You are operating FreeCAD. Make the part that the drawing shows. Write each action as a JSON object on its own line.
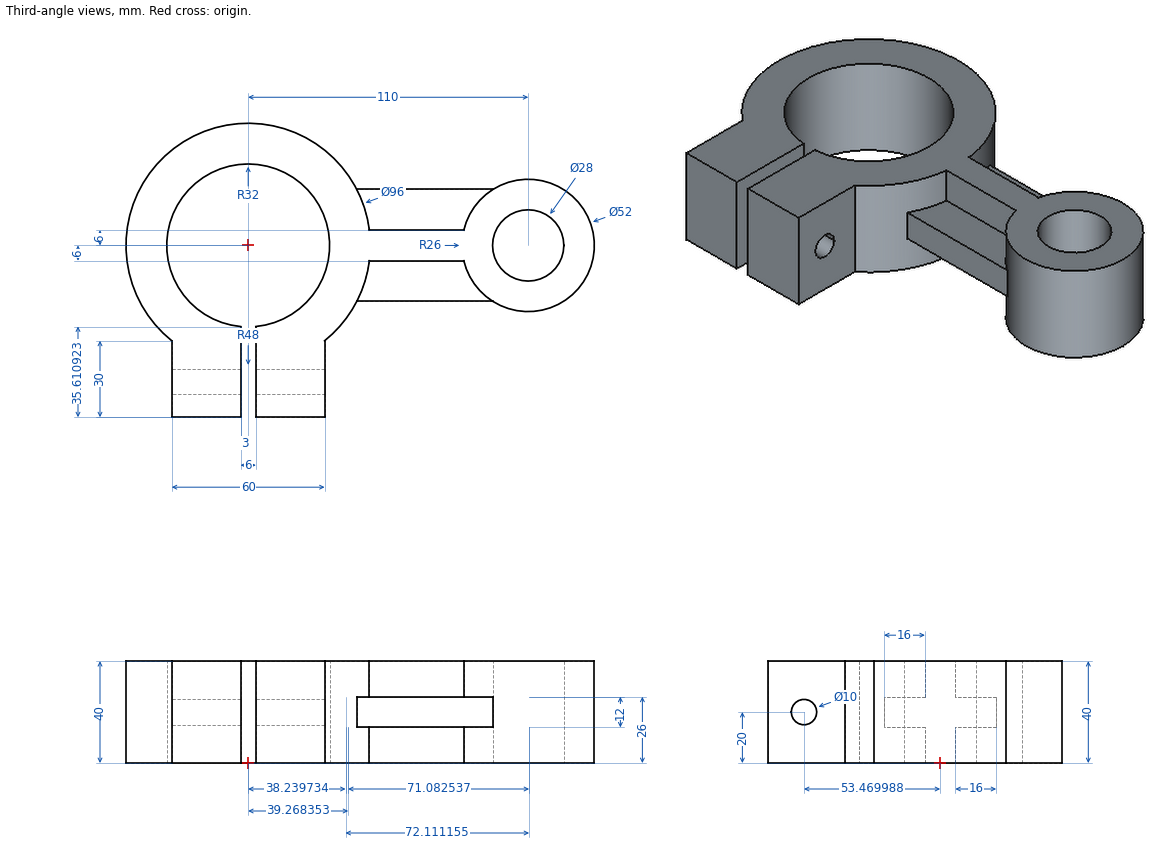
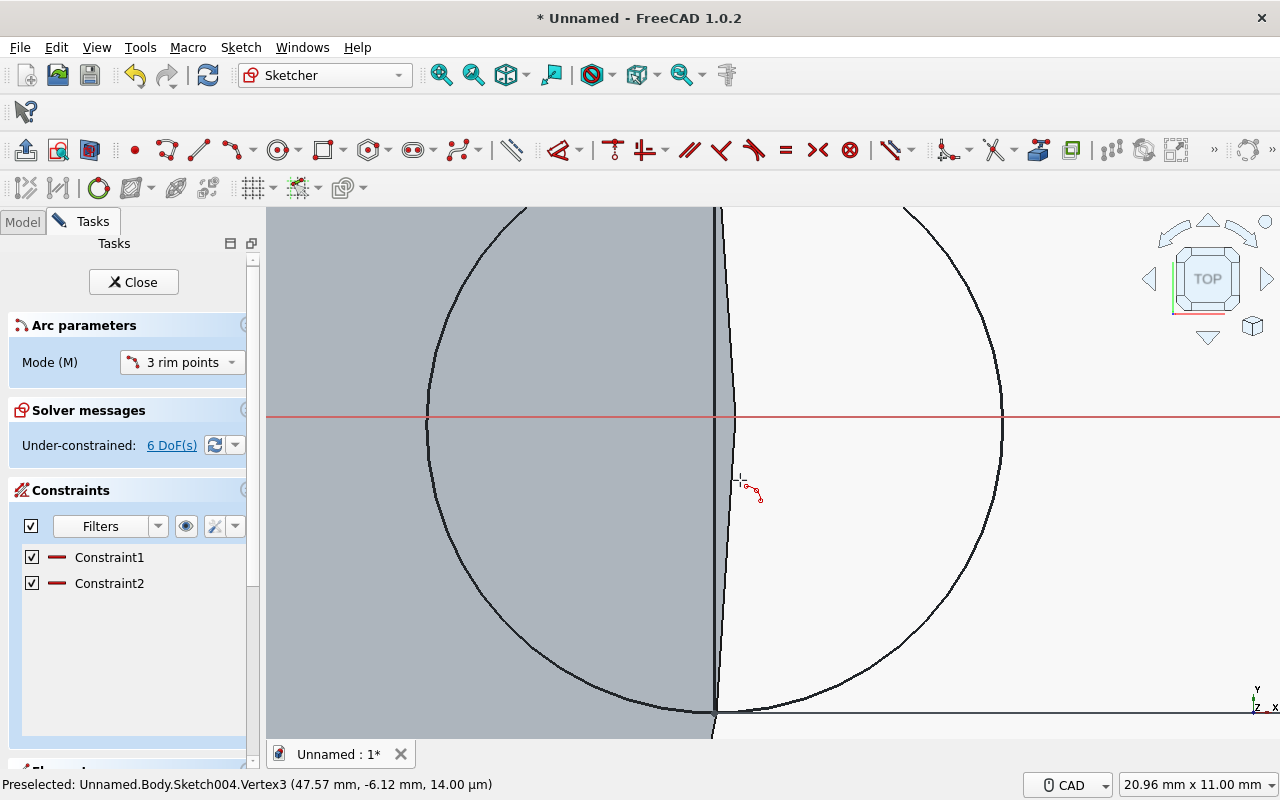
{"action": "left_click", "coordinate": [735, 475]}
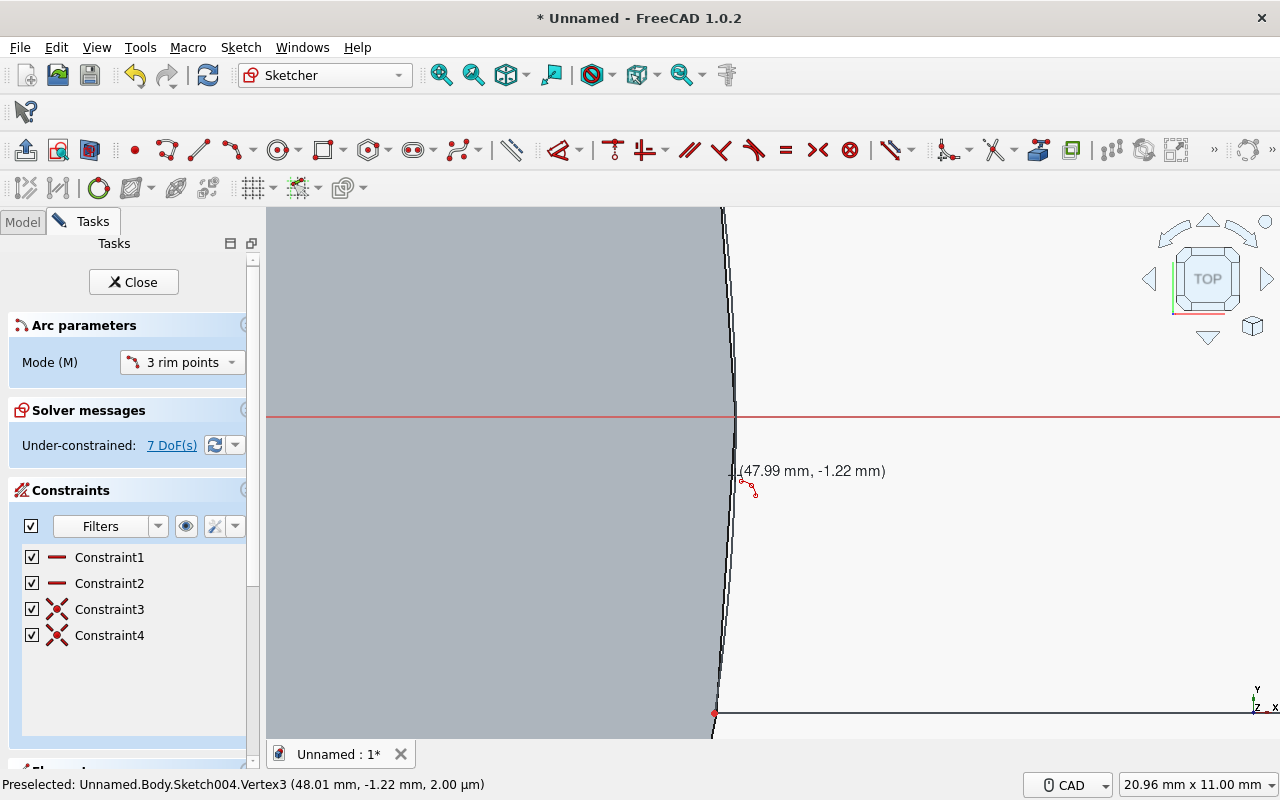
{"action": "scroll", "coordinate": [742, 482], "scroll_direction": "down", "scroll_amount": 10}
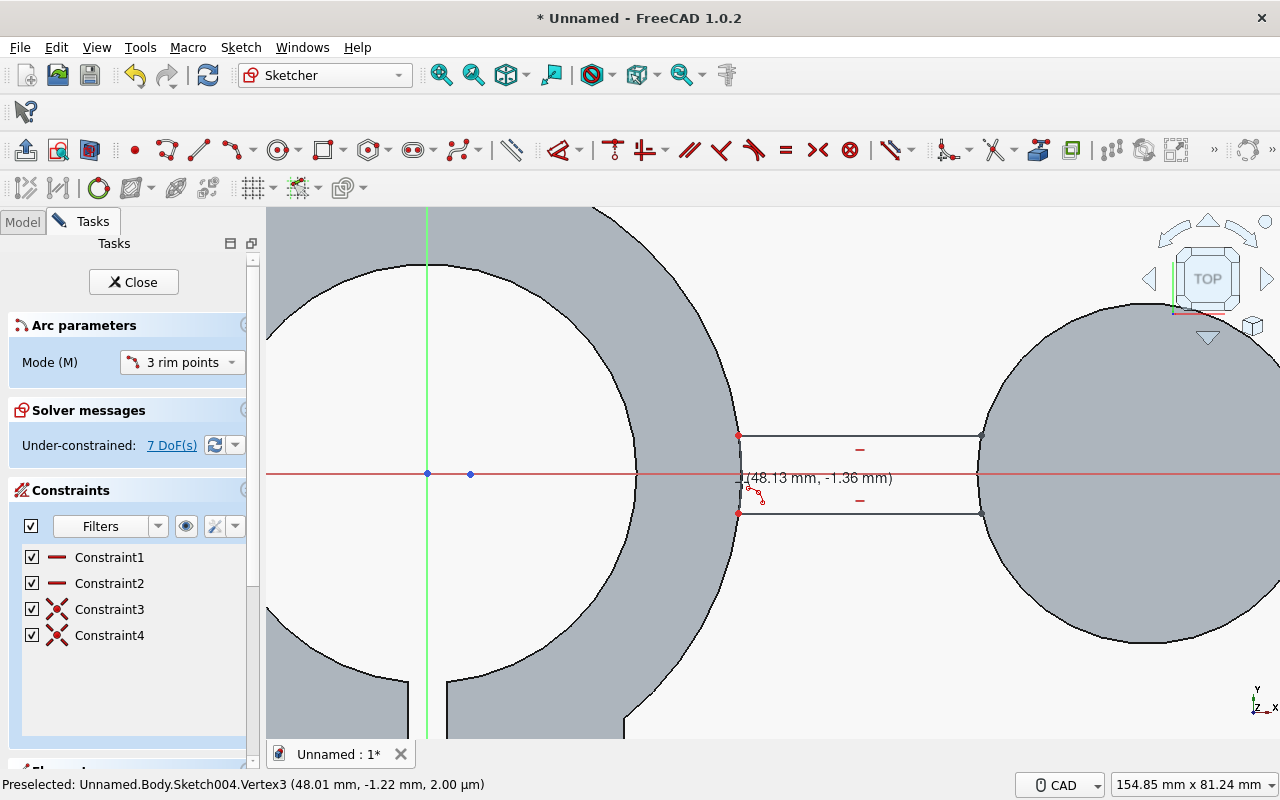
{"action": "left_click", "coordinate": [982, 514]}
{"action": "left_click", "coordinate": [982, 436]}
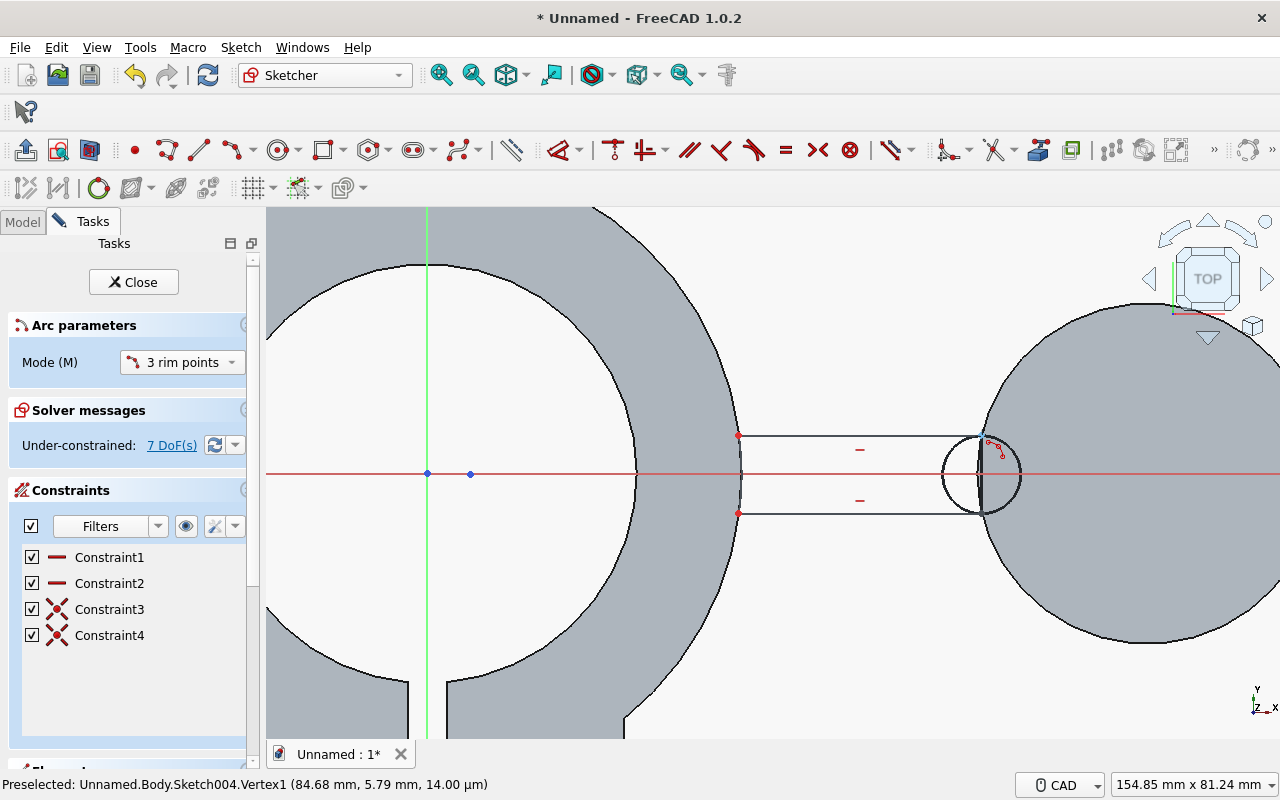
{"action": "scroll", "coordinate": [977, 466], "scroll_direction": "up", "scroll_amount": 7}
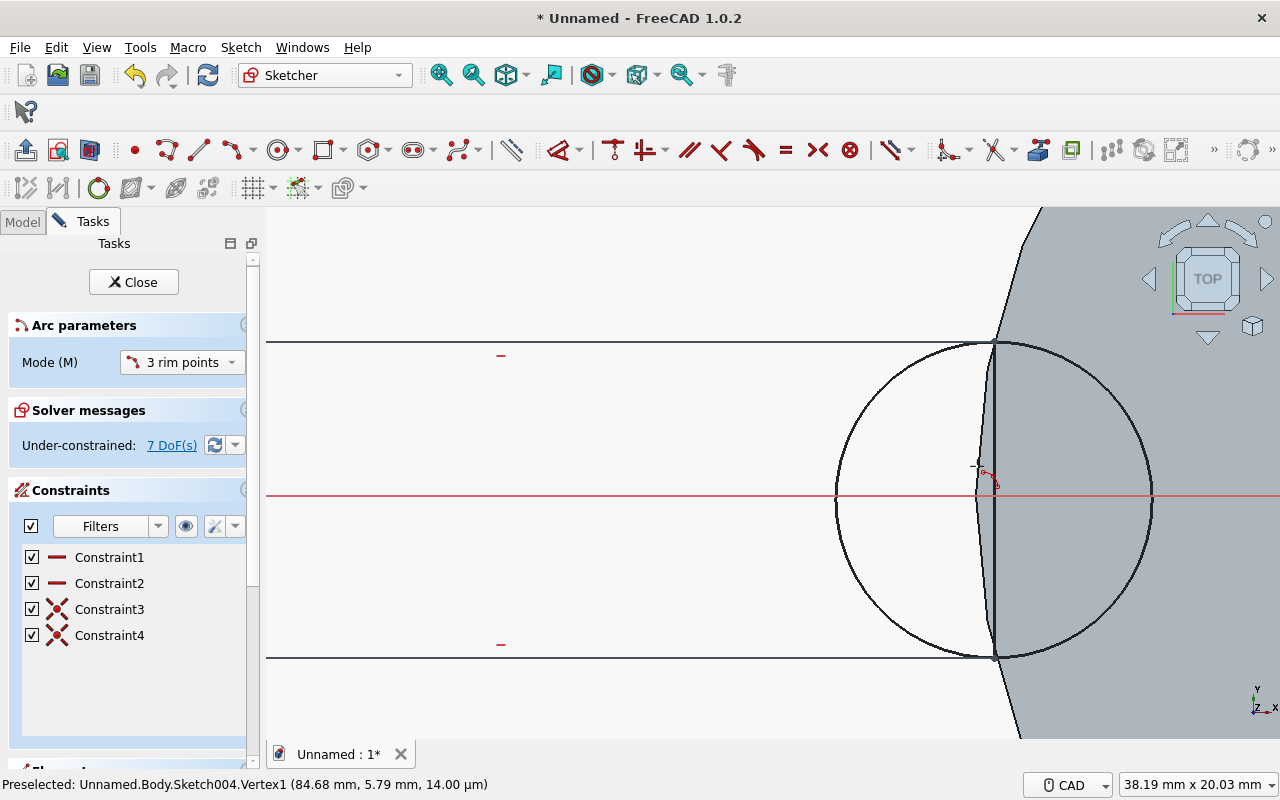
{"action": "left_click", "coordinate": [977, 463]}
{"action": "key", "text": "Escape"}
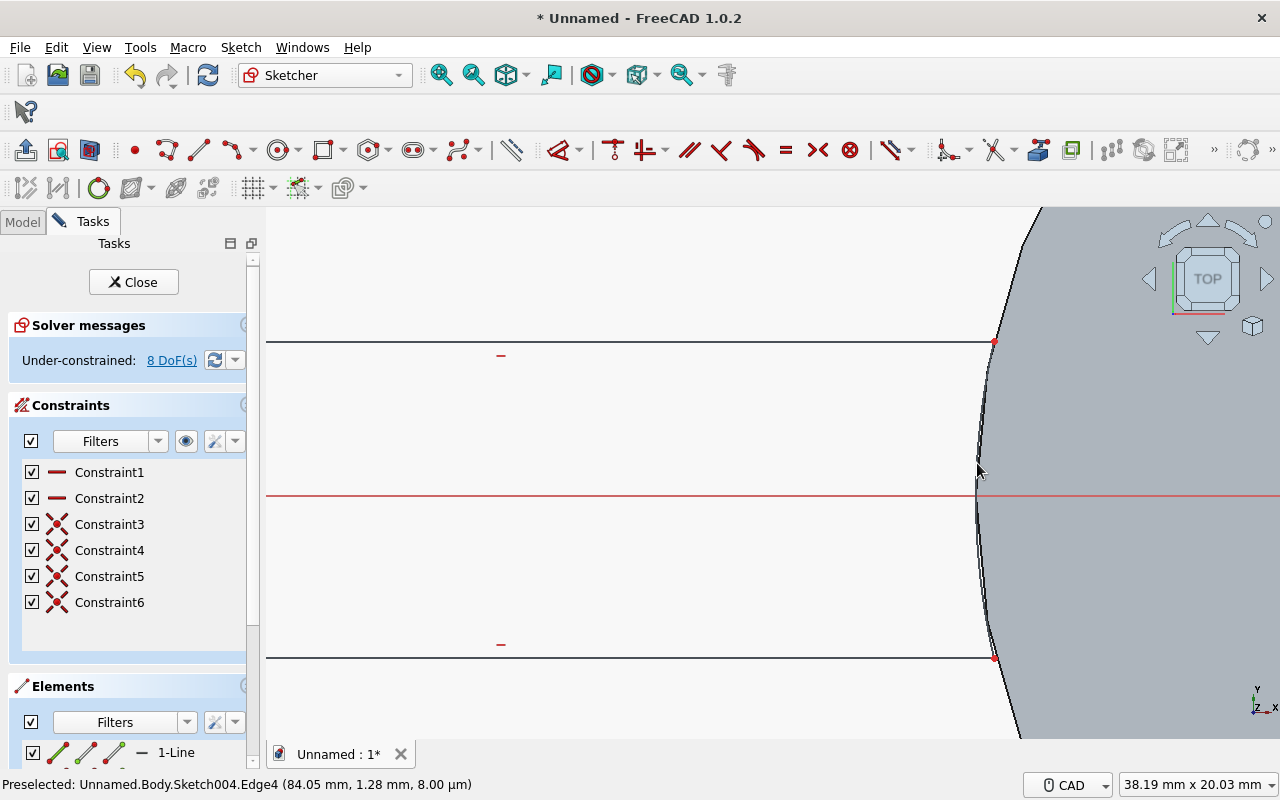
{"action": "scroll", "coordinate": [978, 466], "scroll_direction": "down", "scroll_amount": 7}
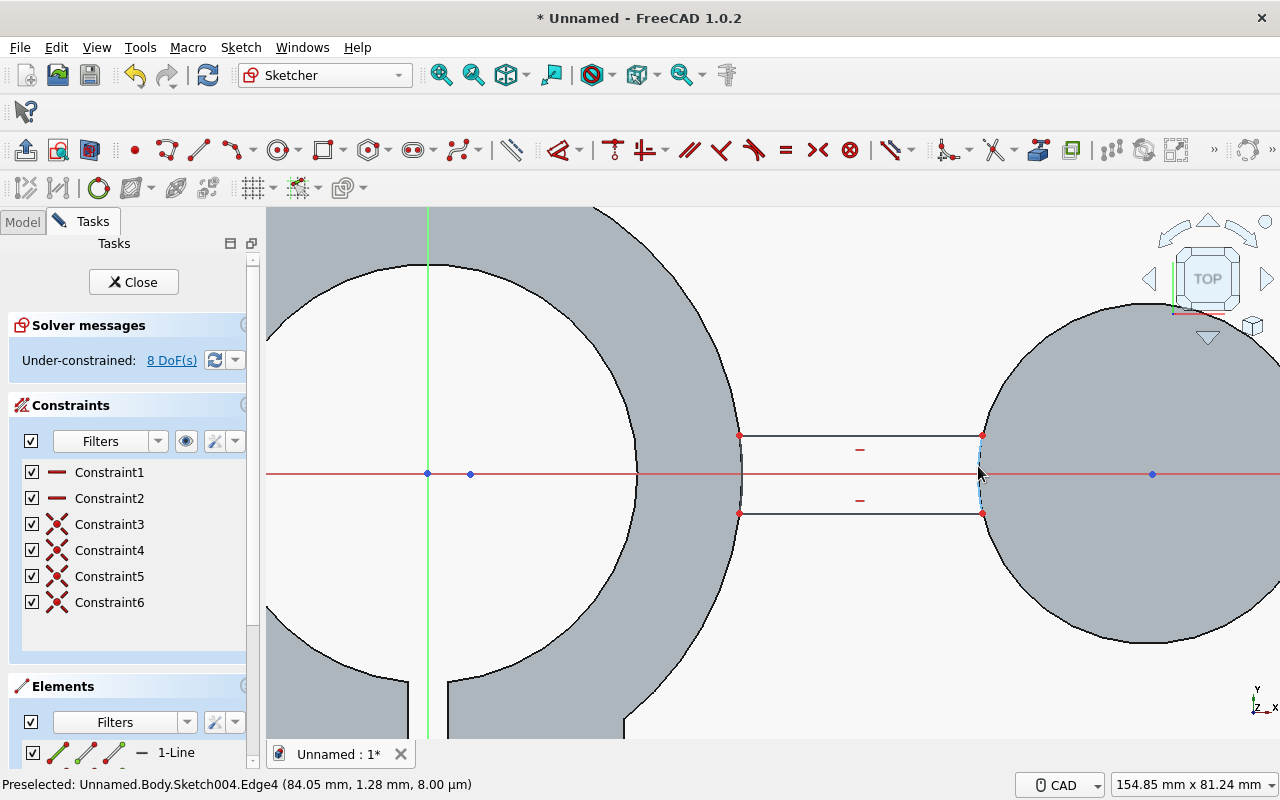
{"action": "left_click_drag", "start_coordinate": [418, 464], "coordinate": [481, 485]}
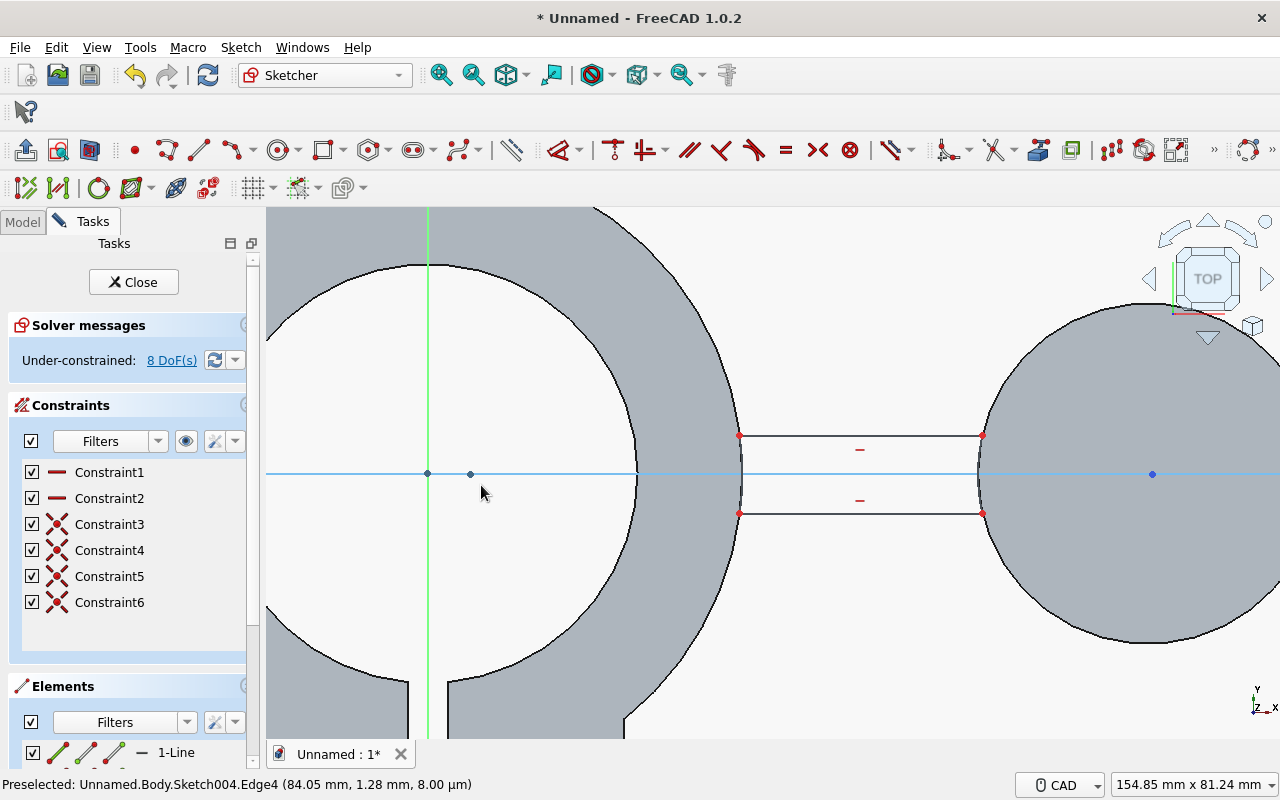
{"action": "left_click", "coordinate": [614, 150]}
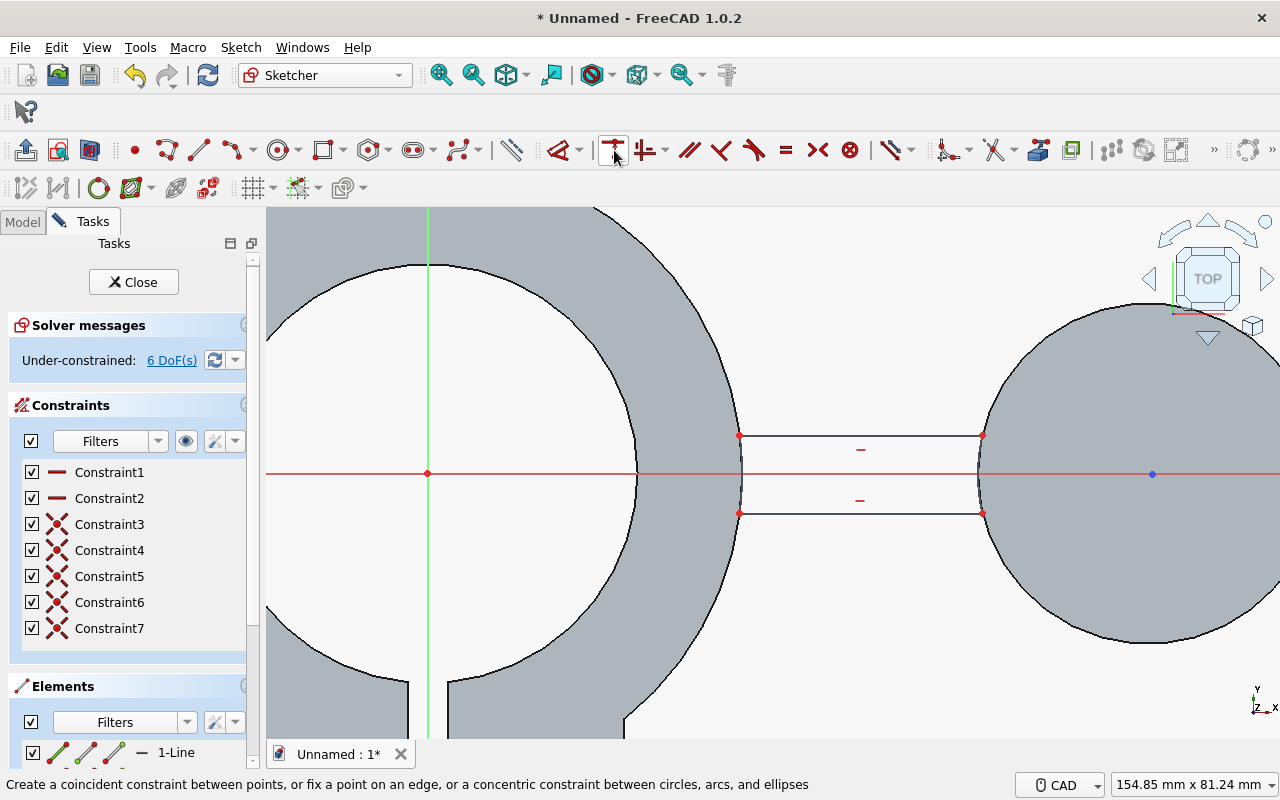
{"action": "scroll", "coordinate": [318, 470], "scroll_direction": "down", "scroll_amount": 1}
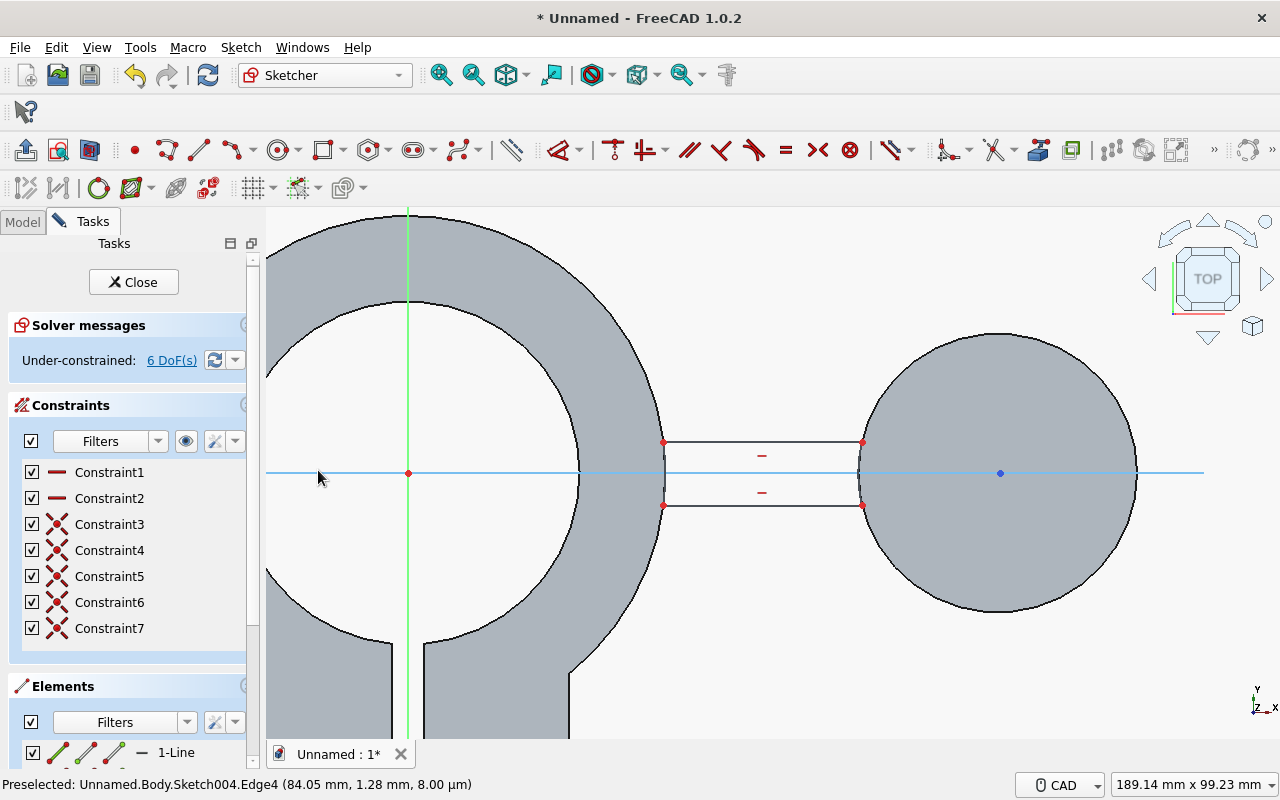
{"action": "left_click", "coordinate": [1001, 474]}